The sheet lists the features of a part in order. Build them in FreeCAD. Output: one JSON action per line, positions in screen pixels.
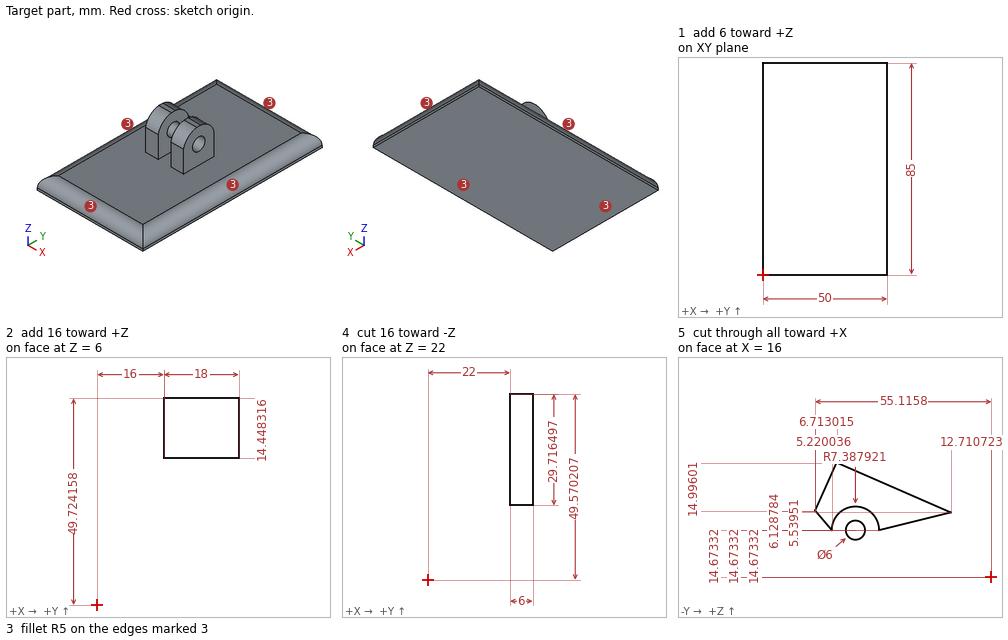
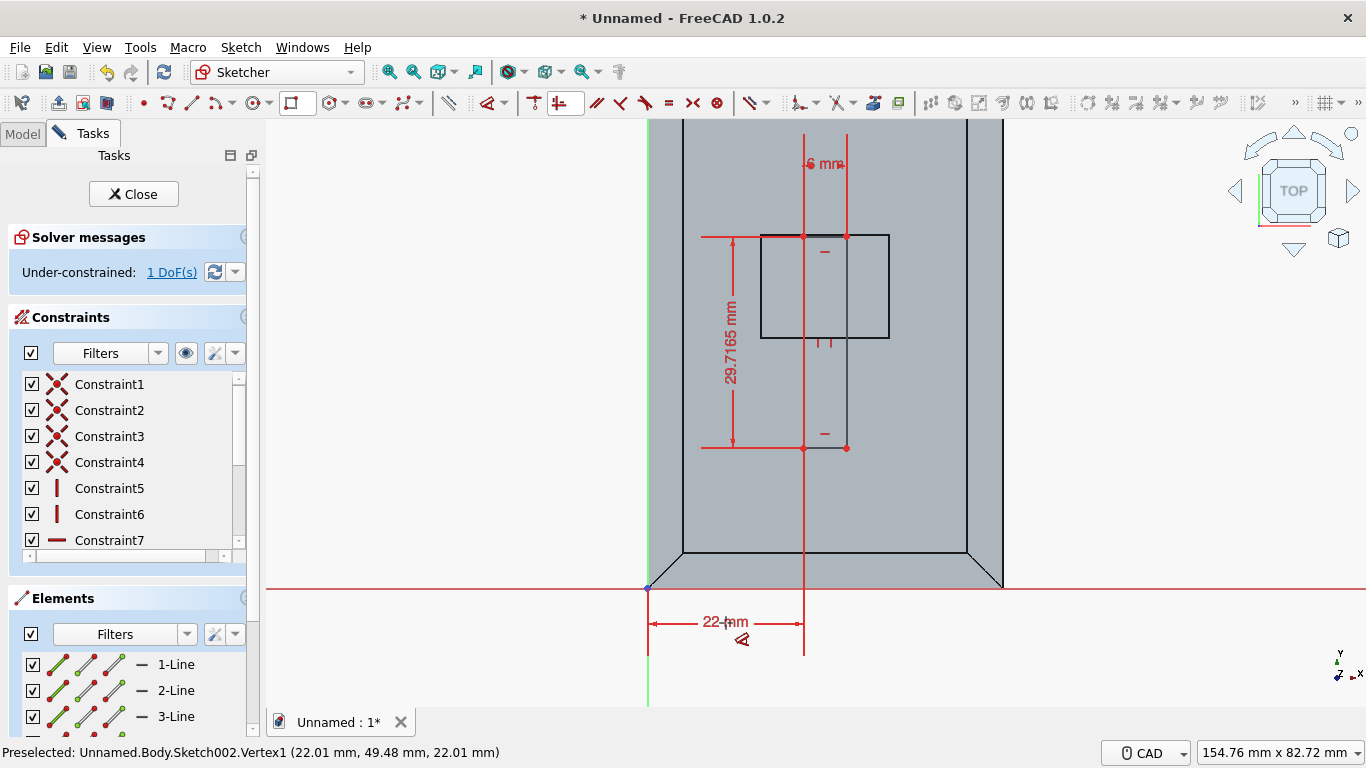
{"action": "left_click", "coordinate": [804, 237]}
{"action": "left_click", "coordinate": [614, 413]}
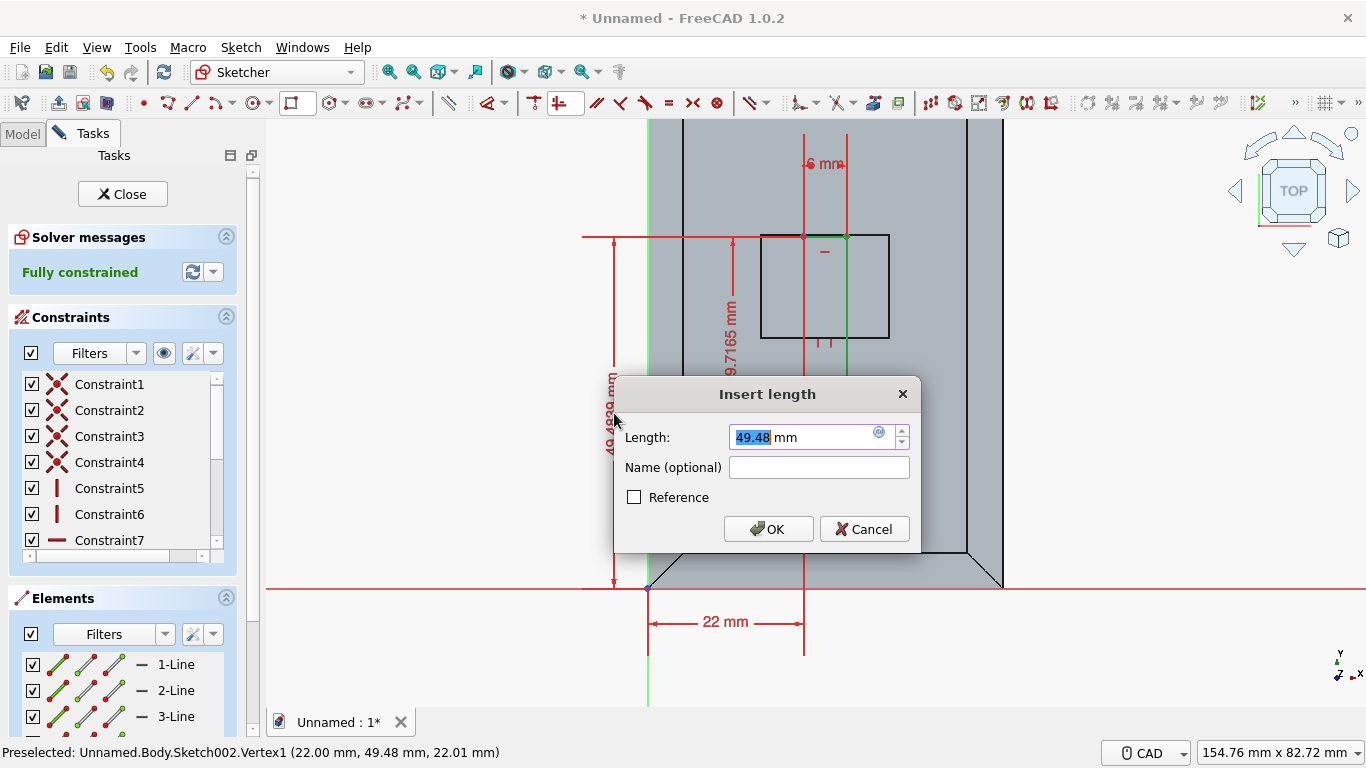
{"action": "type", "text": "49.570207"}
{"action": "key", "text": "Return"}
{"action": "key", "text": "Escape"}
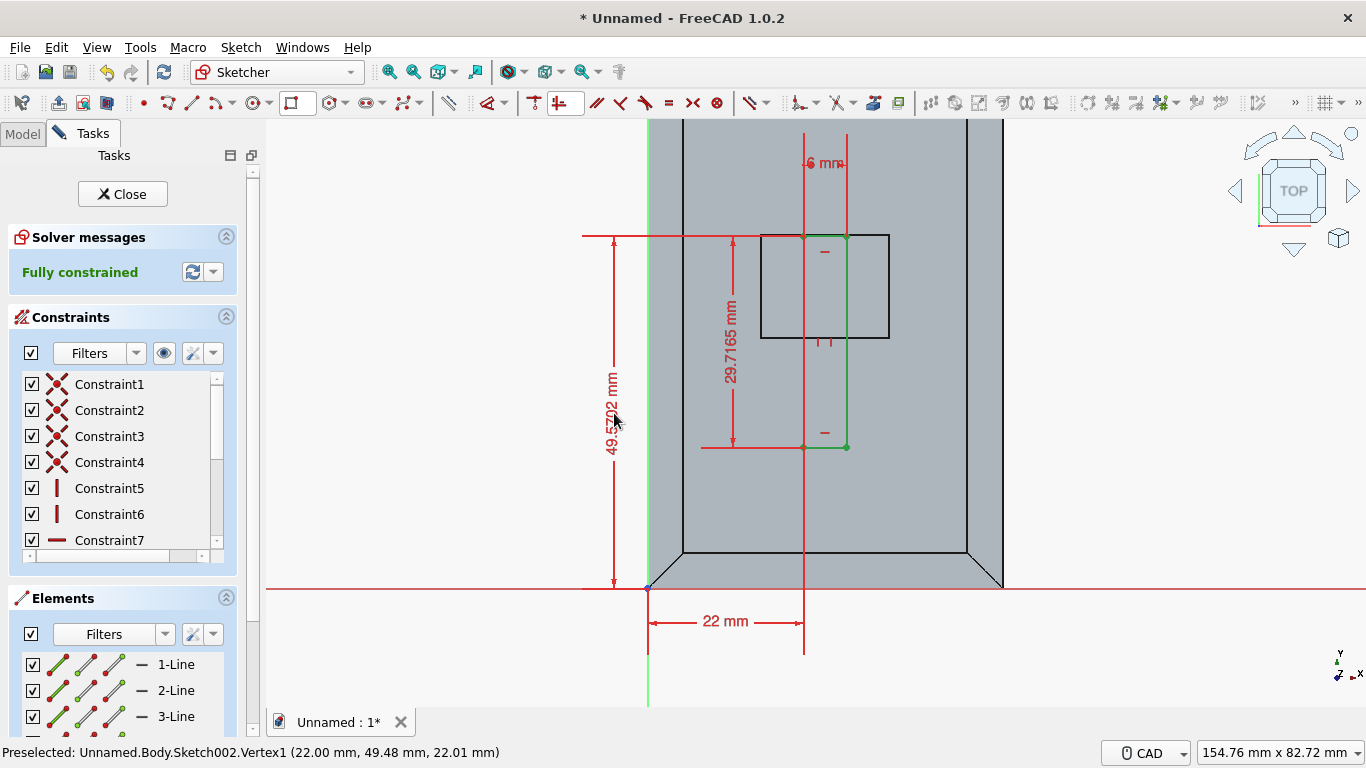
{"action": "left_click", "coordinate": [123, 194]}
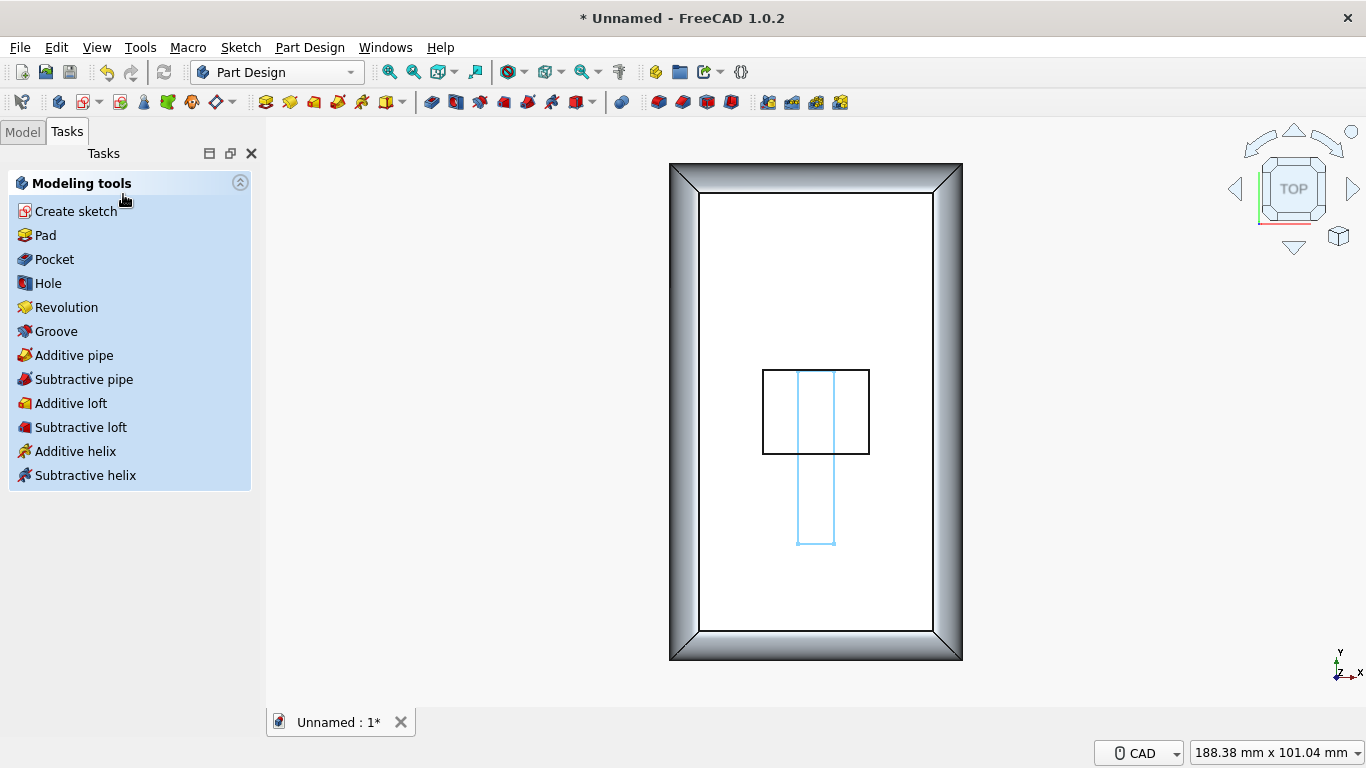
{"action": "left_click", "coordinate": [432, 102]}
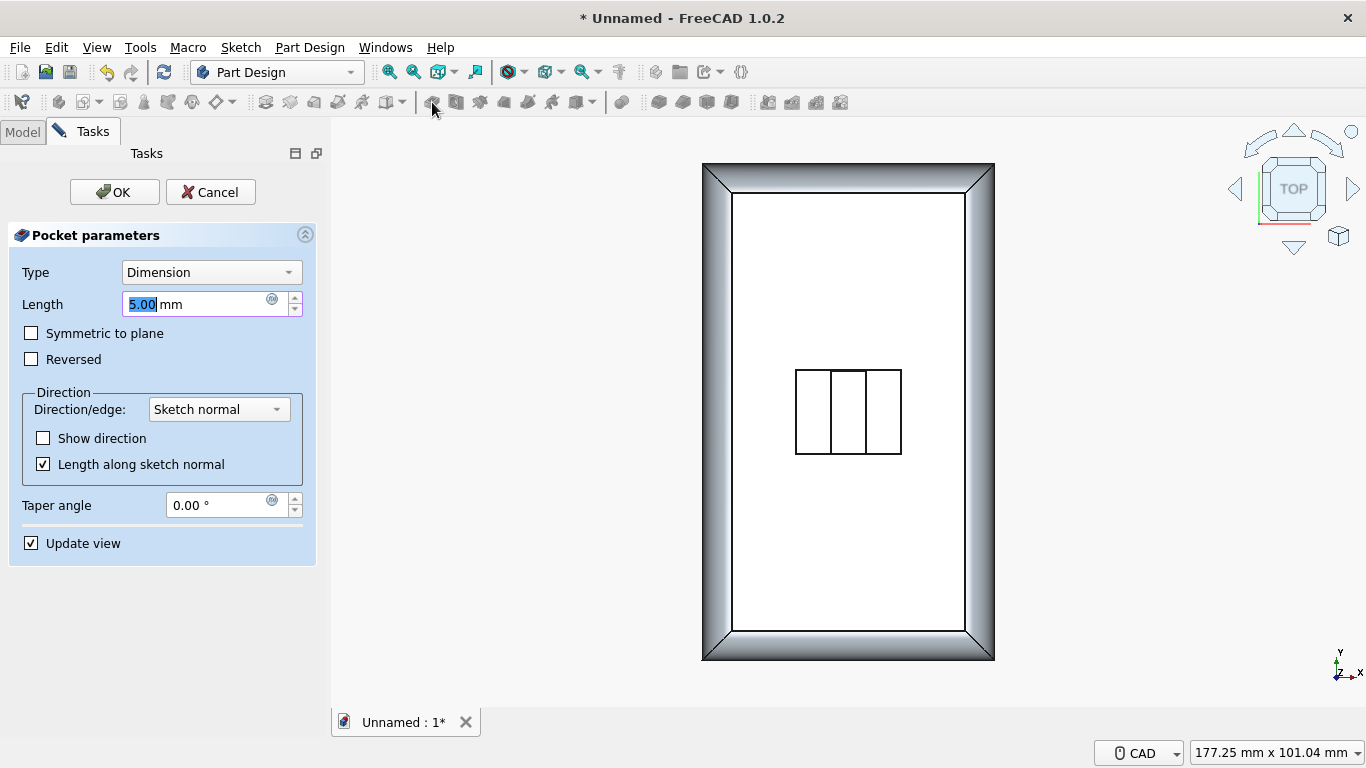
{"action": "type", "text": "16"}
{"action": "key", "text": "Tab"}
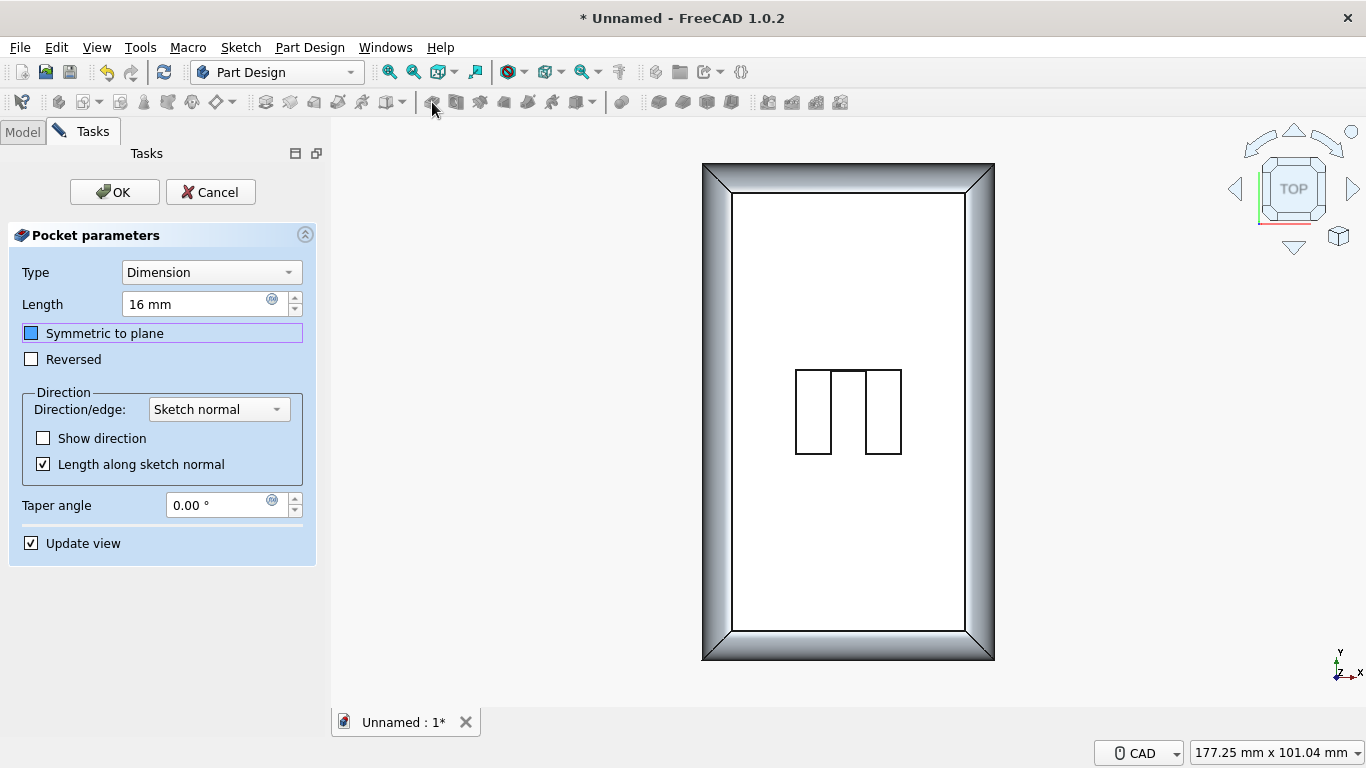
{"action": "left_click", "coordinate": [115, 192]}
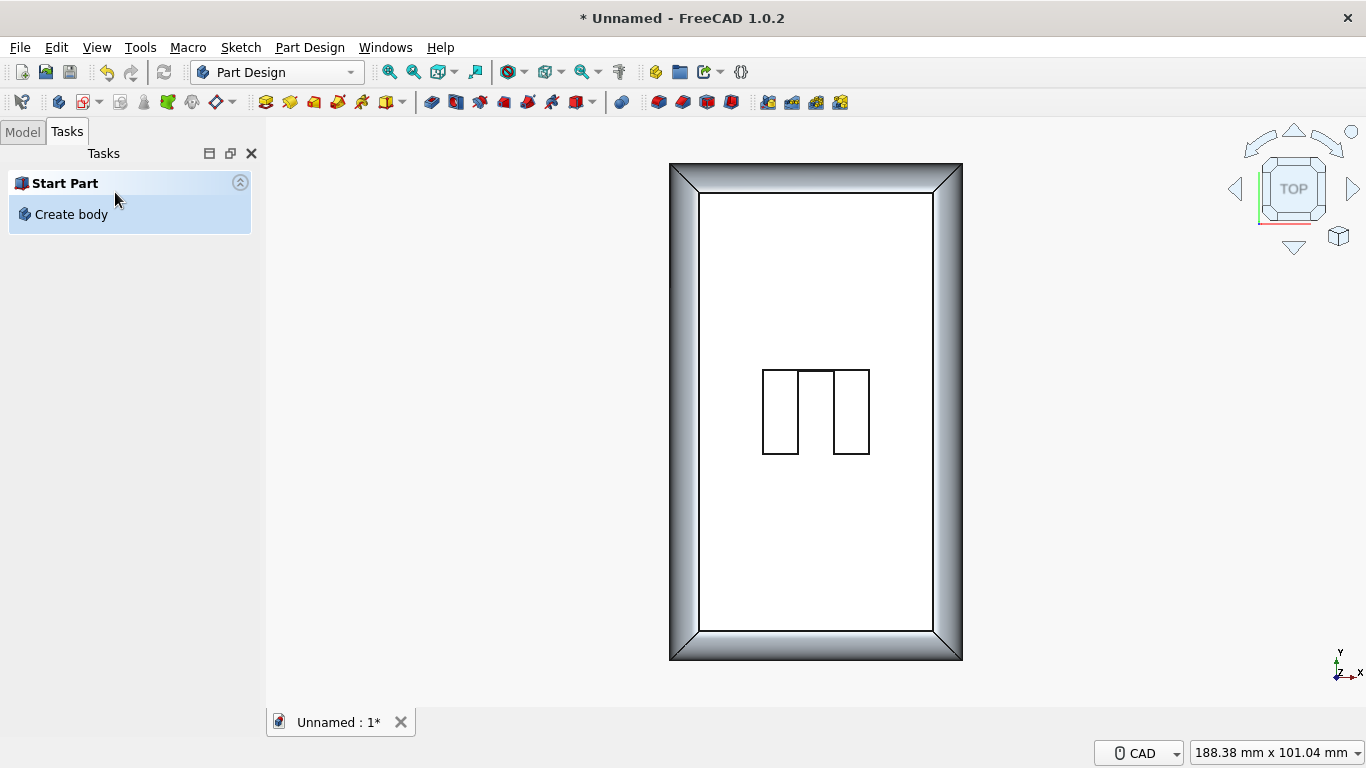
{"action": "key", "text": "6"}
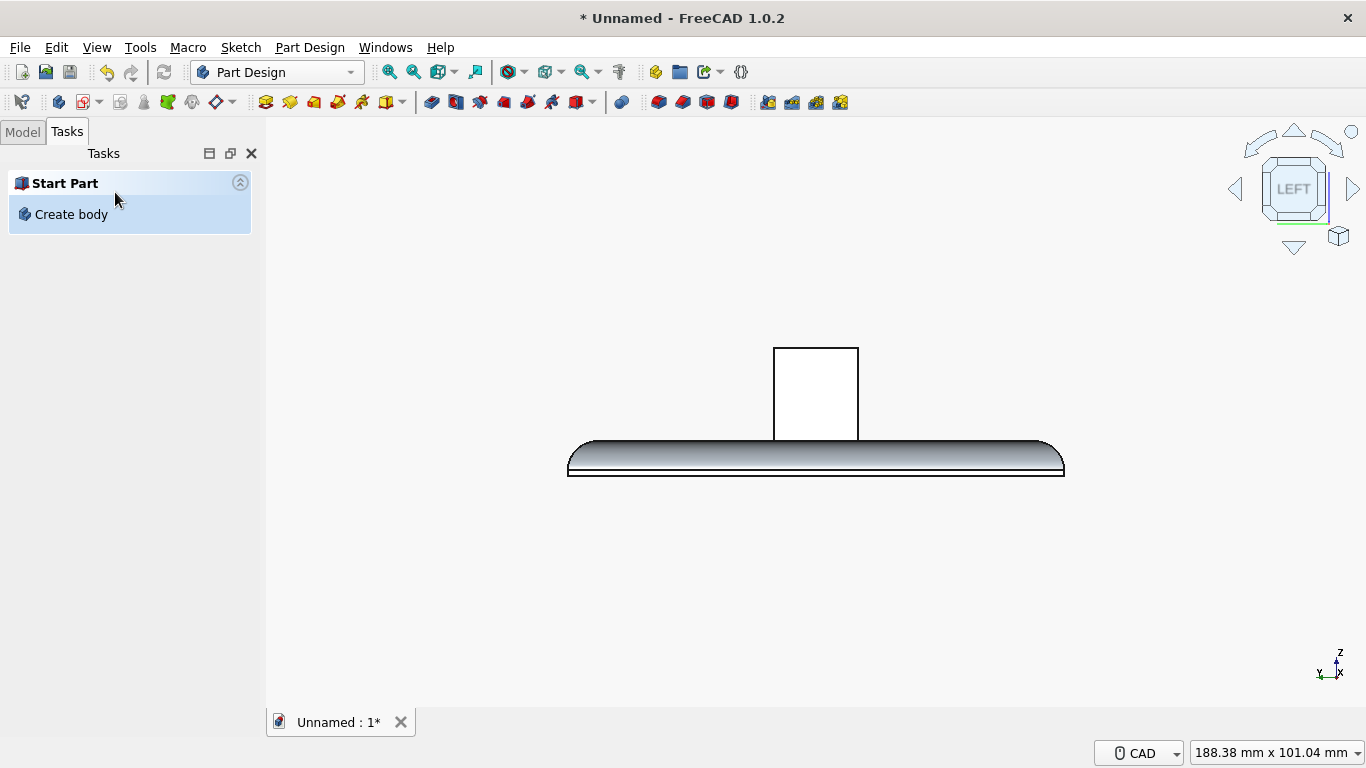
{"action": "left_click", "coordinate": [816, 393]}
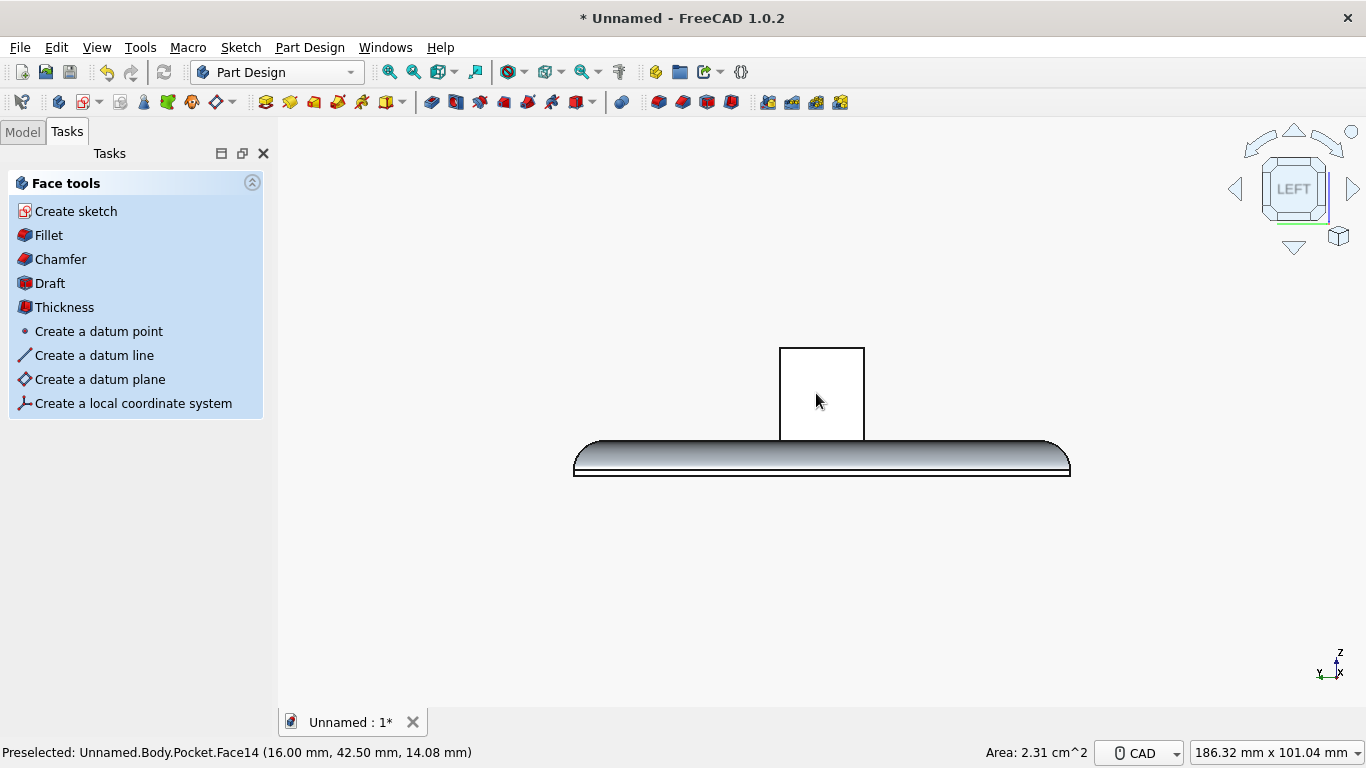
{"action": "left_click", "coordinate": [84, 102]}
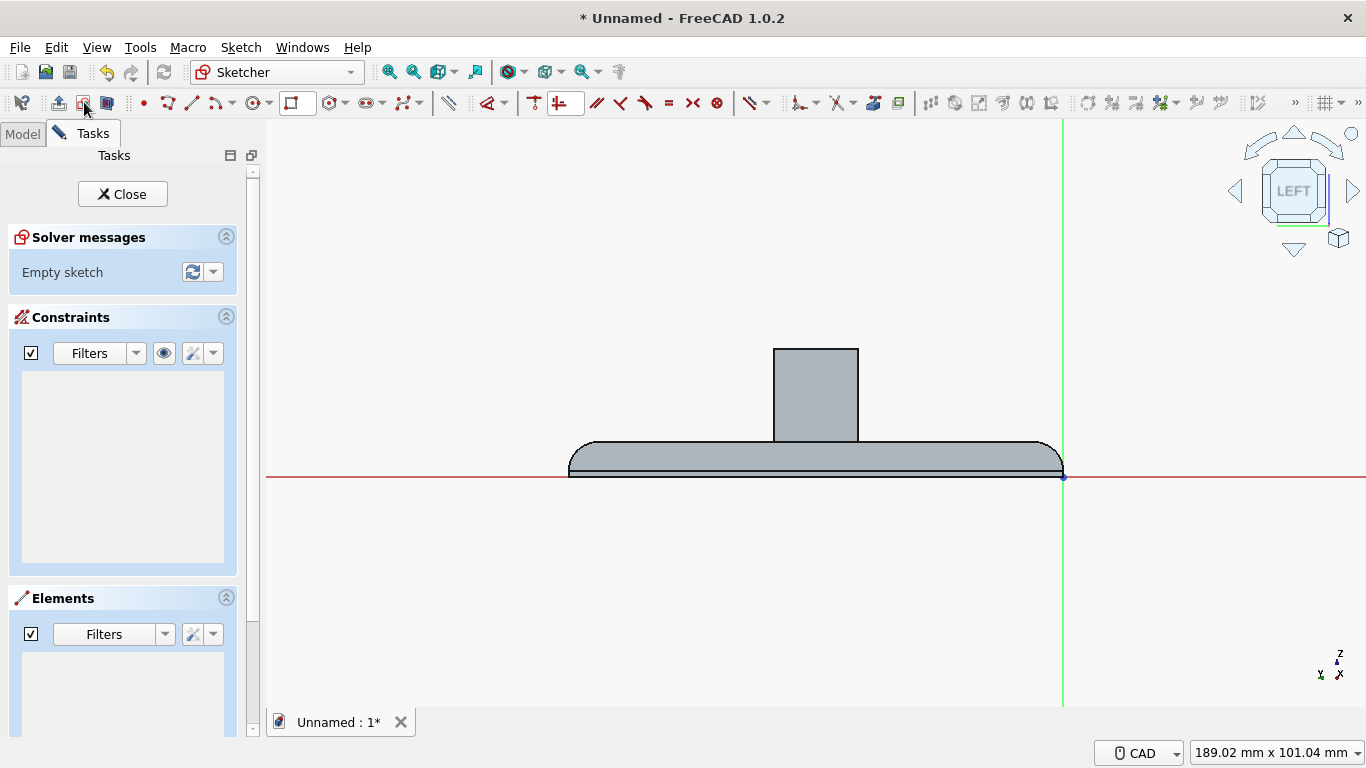
{"action": "scroll", "coordinate": [1092, 324], "scroll_direction": "up", "scroll_amount": 3}